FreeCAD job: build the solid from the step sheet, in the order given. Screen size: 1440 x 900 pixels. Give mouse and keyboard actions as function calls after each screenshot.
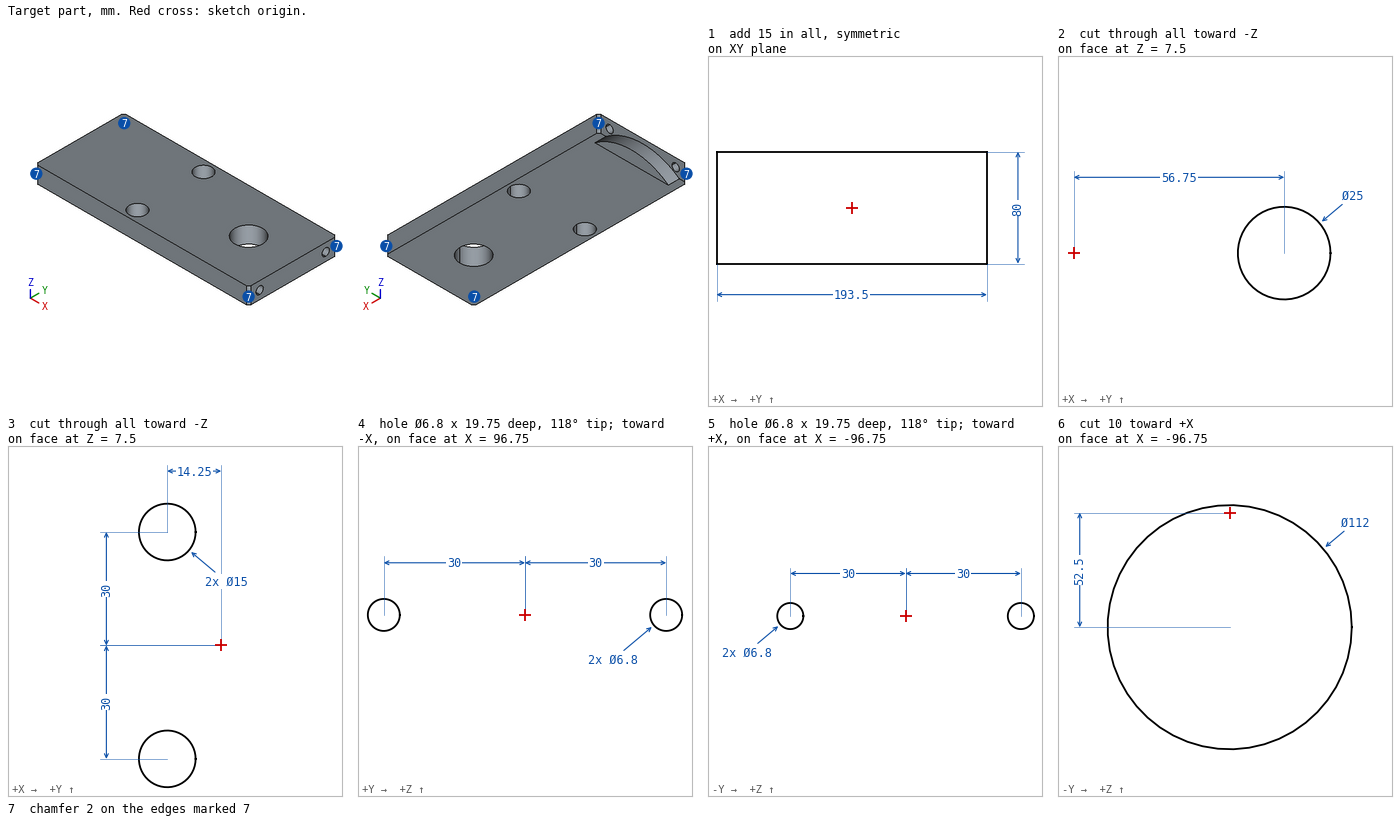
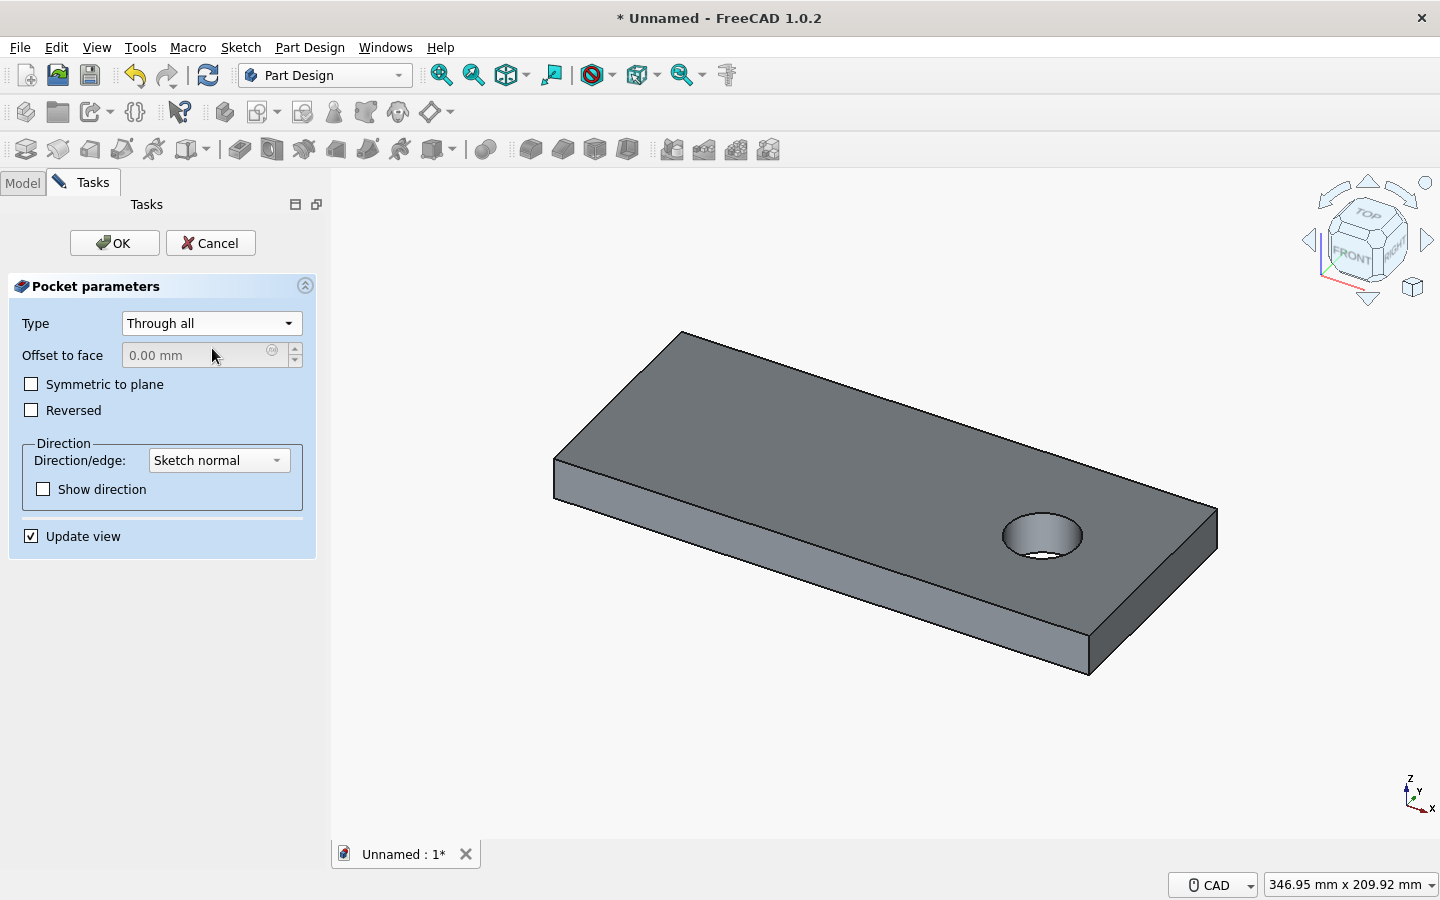
click(115, 243)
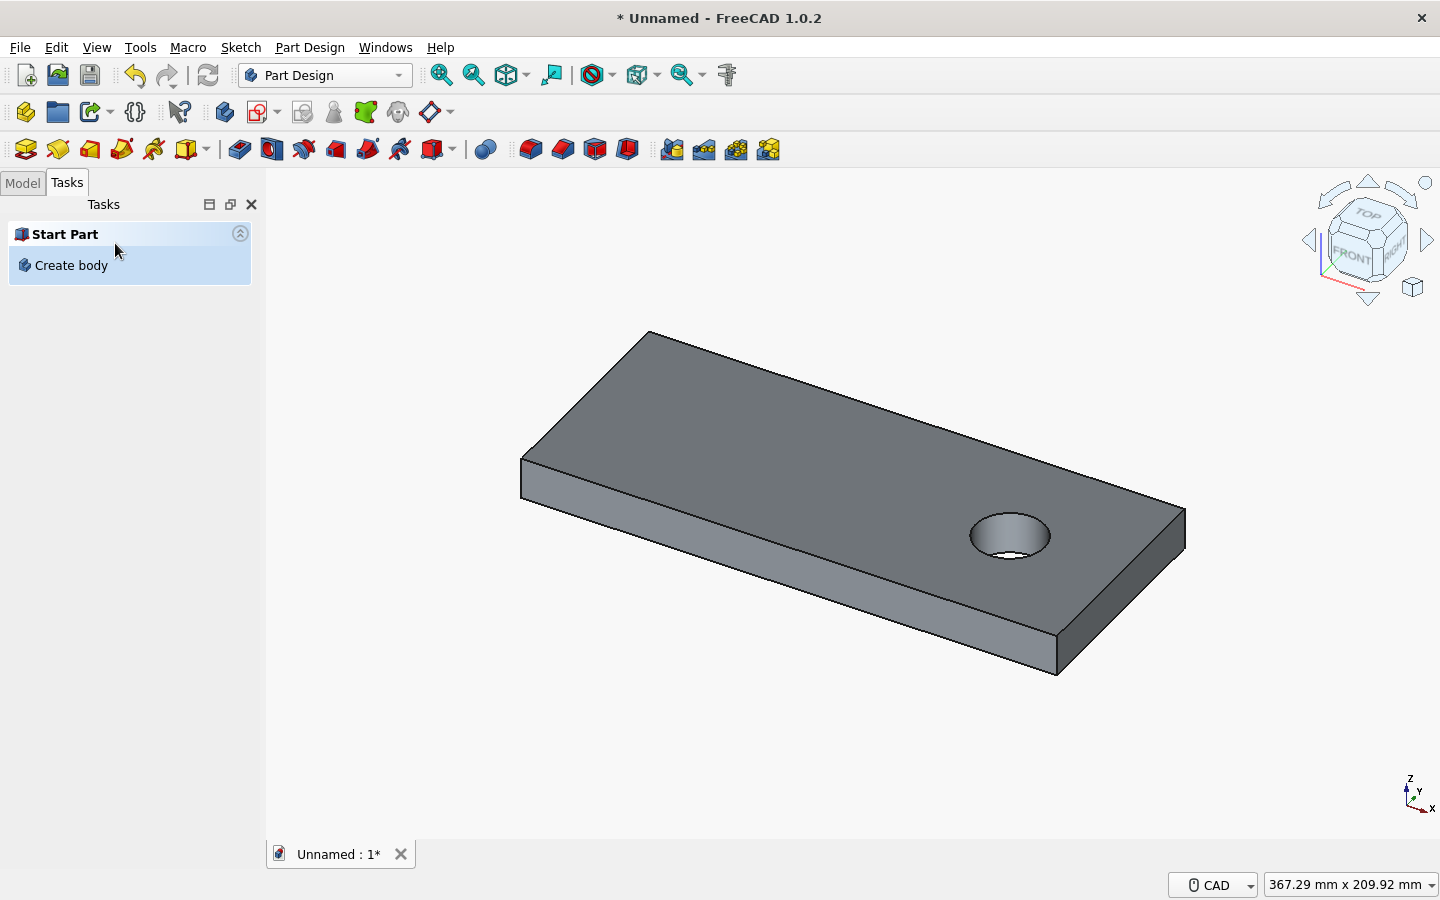
click(853, 483)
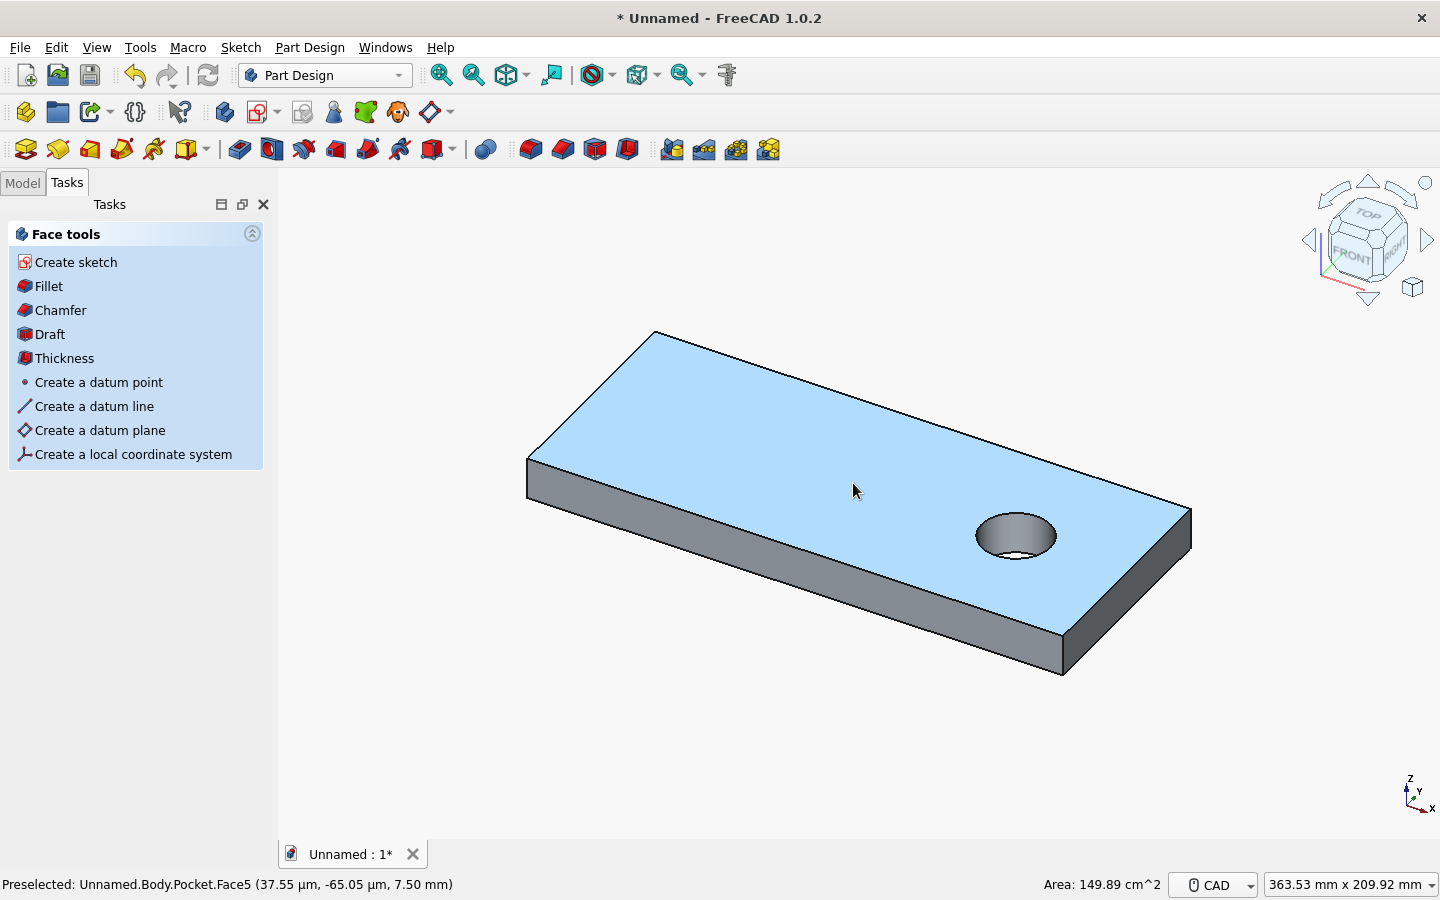
click(258, 112)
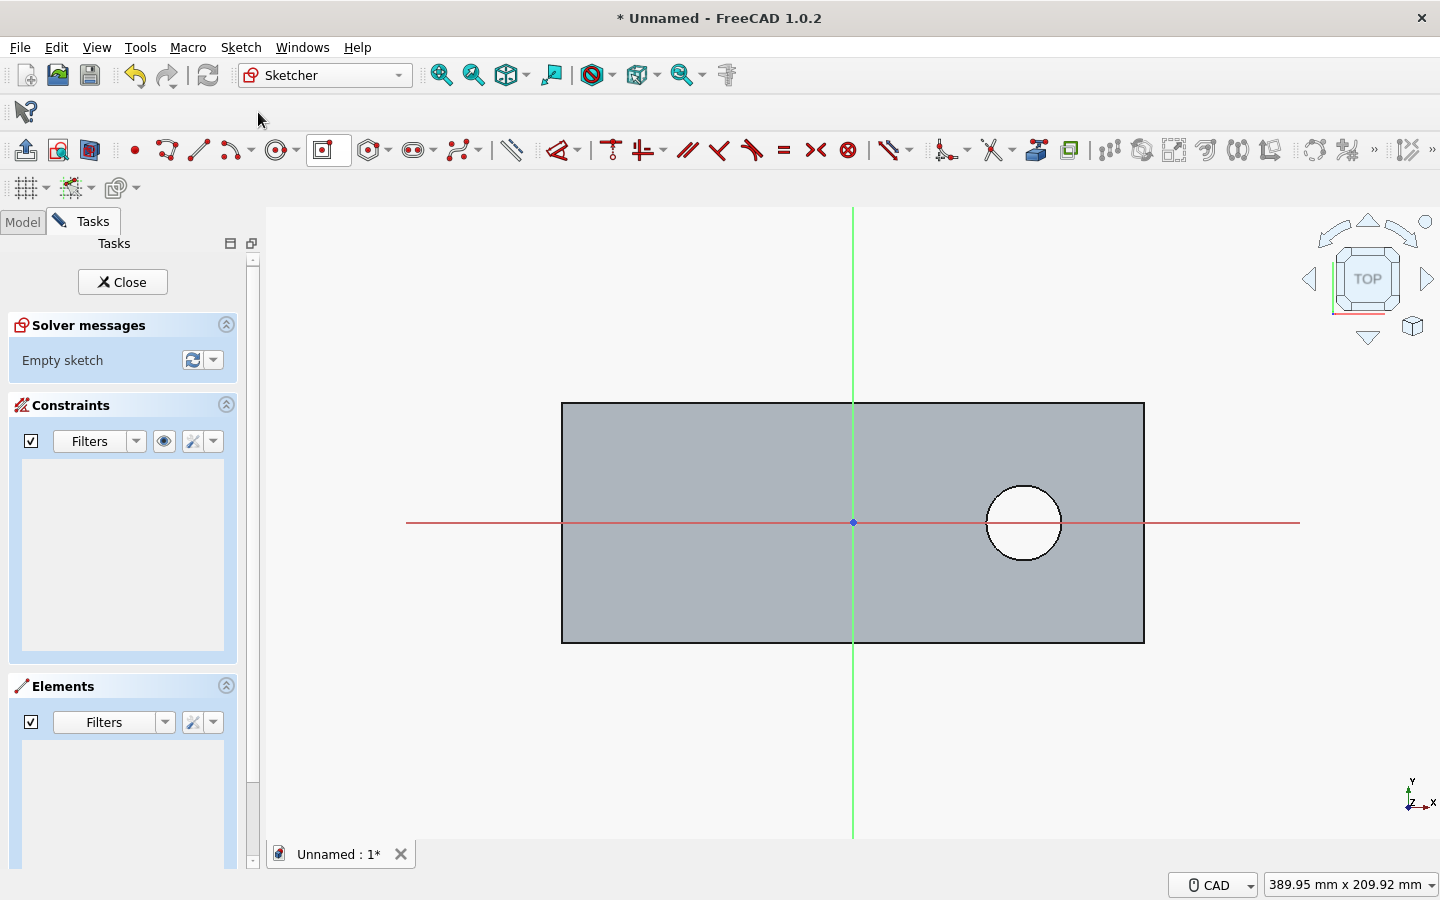
scroll(864, 523, up, 3)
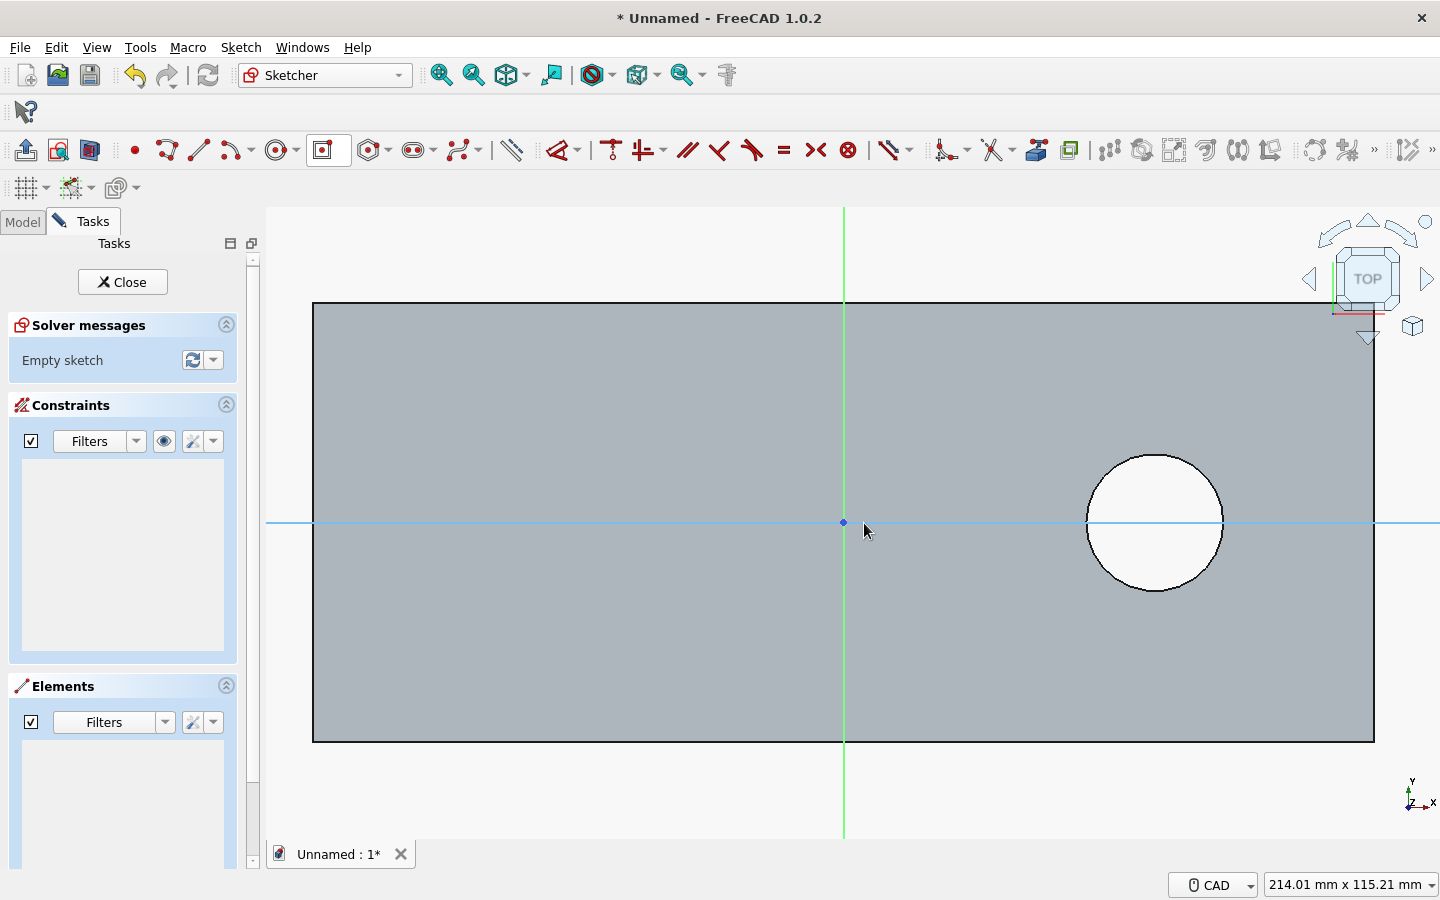
key(g)
key(c)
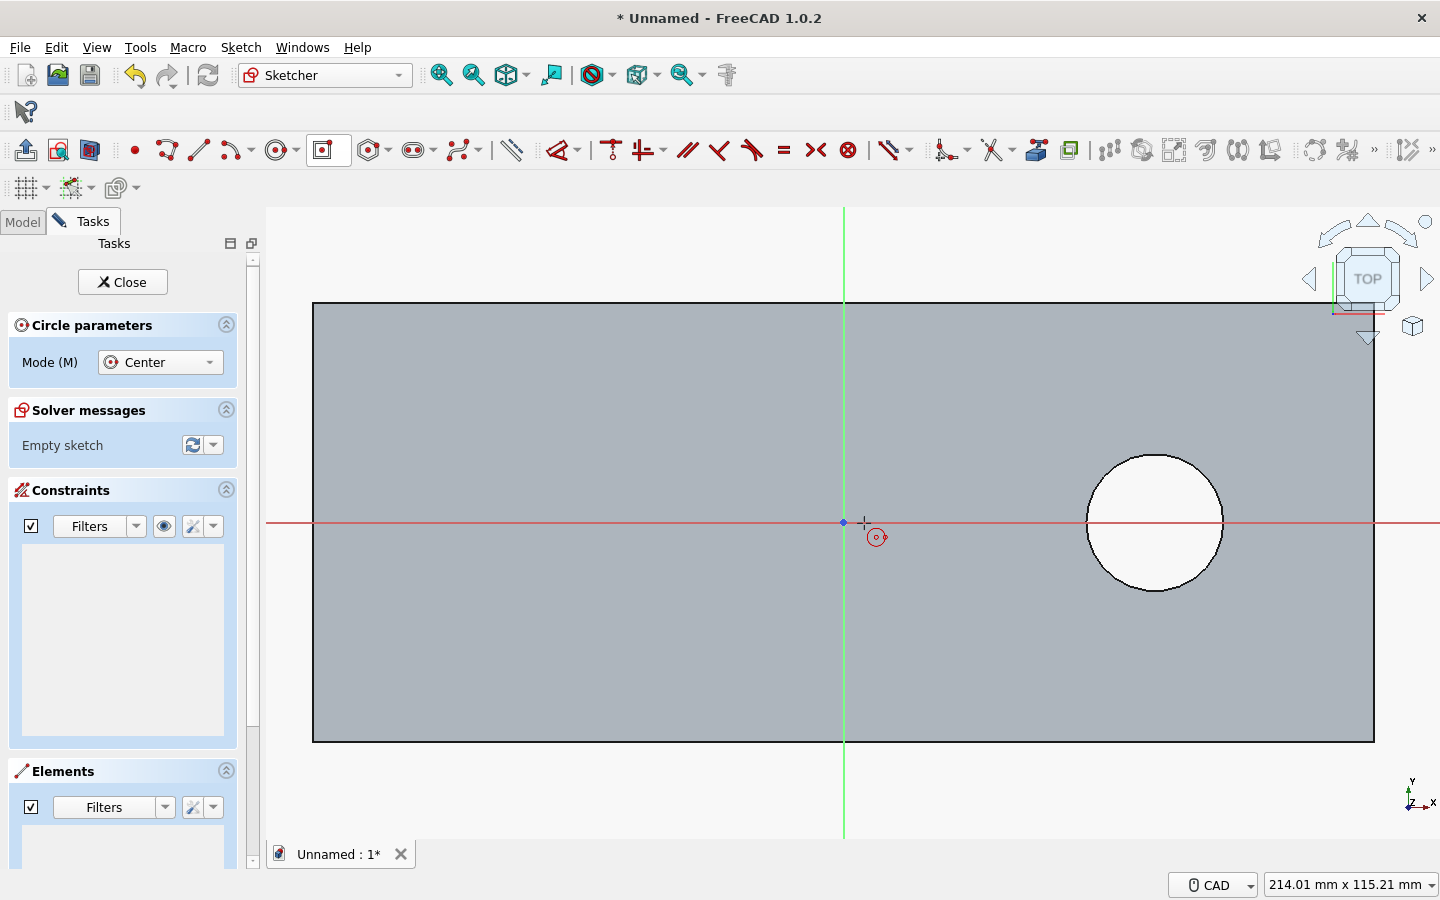
click(765, 358)
move(794, 329)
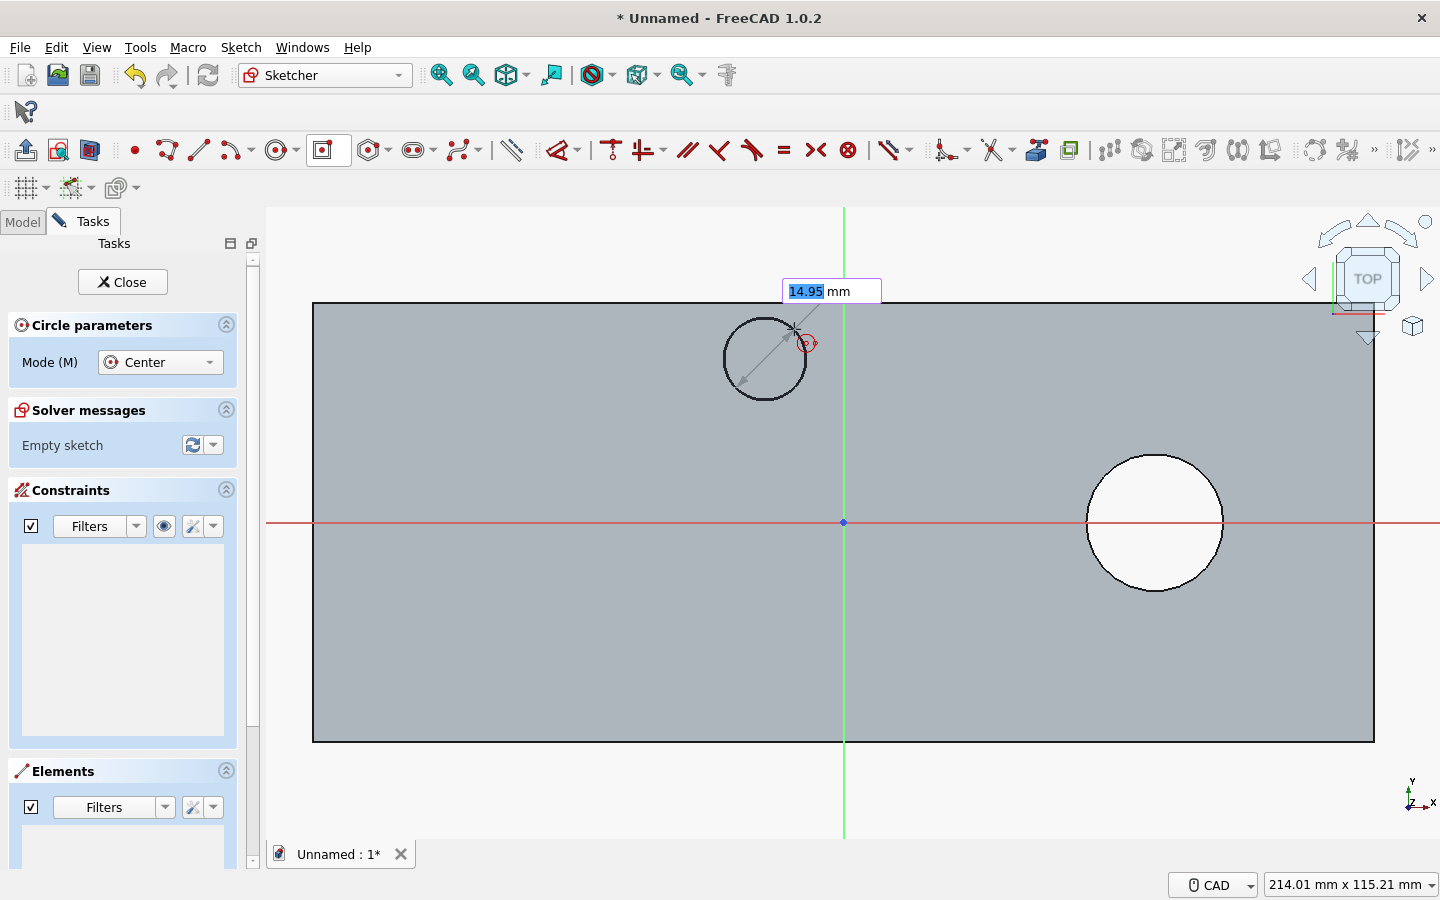
text(15)
key(Return)